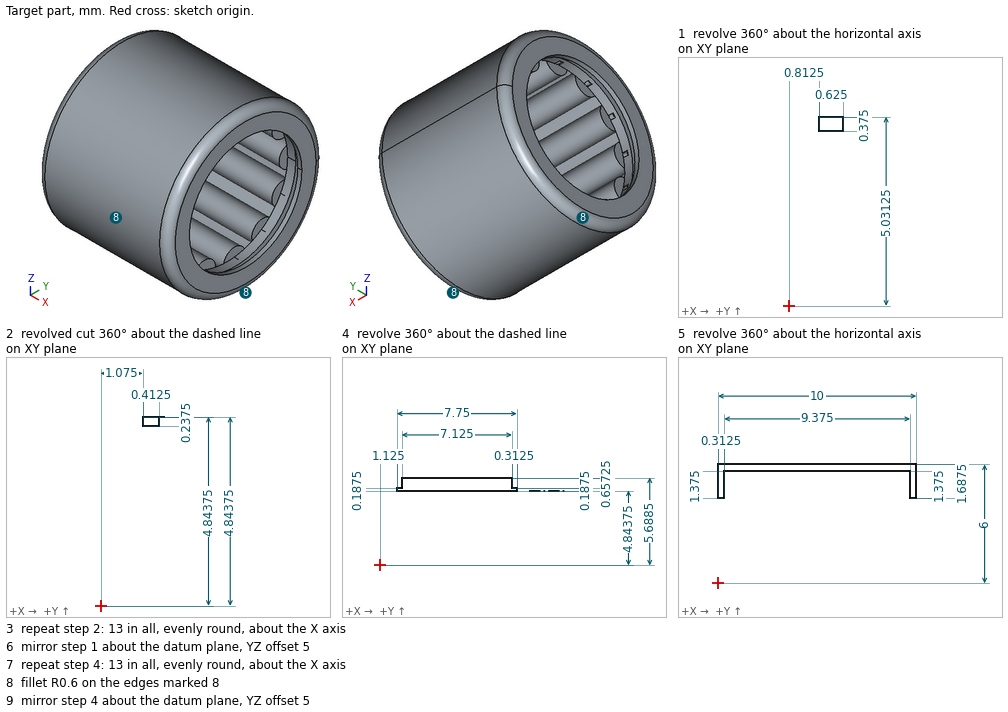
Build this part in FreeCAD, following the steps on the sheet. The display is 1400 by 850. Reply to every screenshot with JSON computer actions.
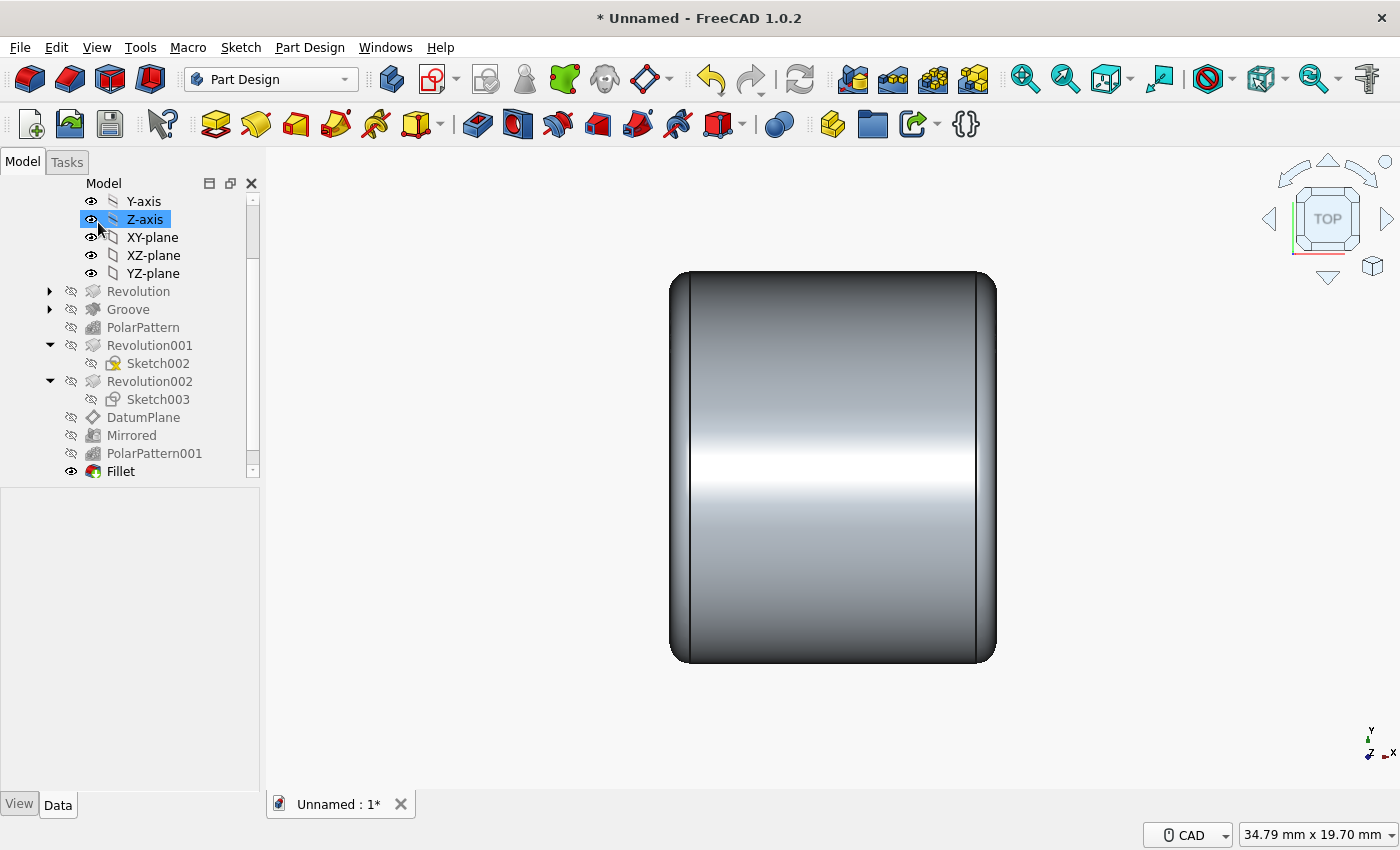
{"action": "scroll", "coordinate": [160, 341], "scroll_direction": "down", "scroll_amount": 3}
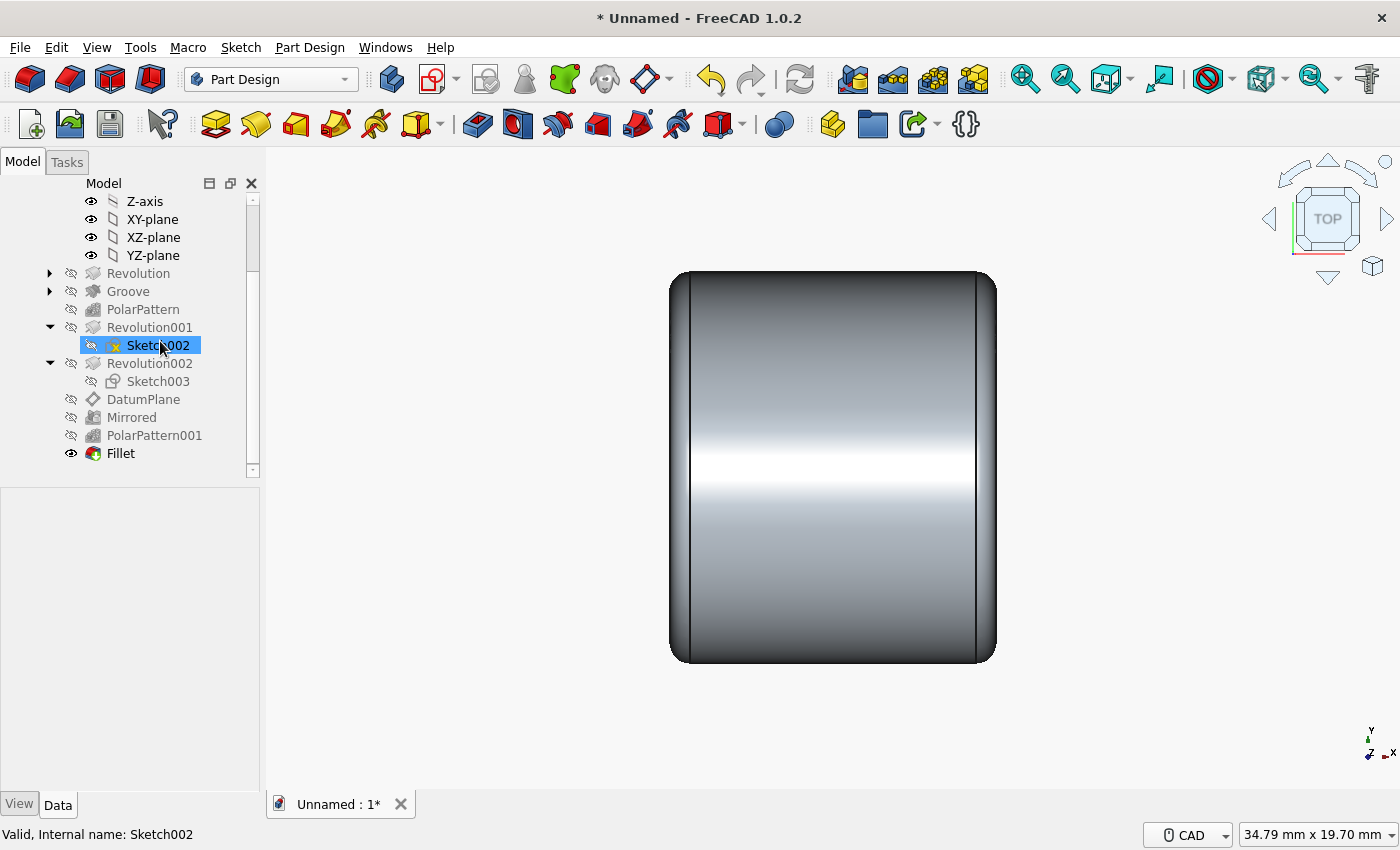
{"action": "scroll", "coordinate": [160, 323], "scroll_direction": "up", "scroll_amount": 15}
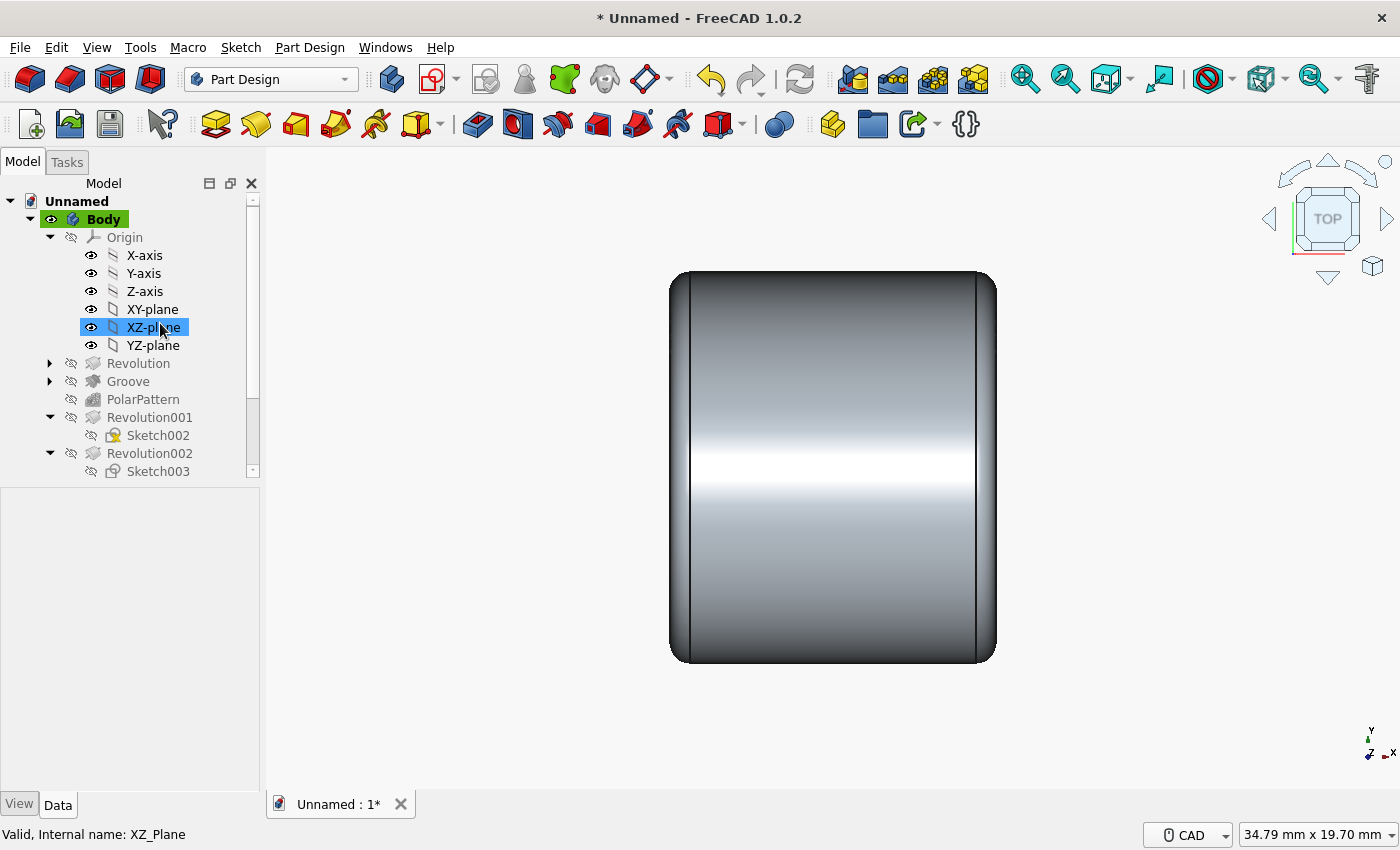
{"action": "left_click", "coordinate": [136, 345]}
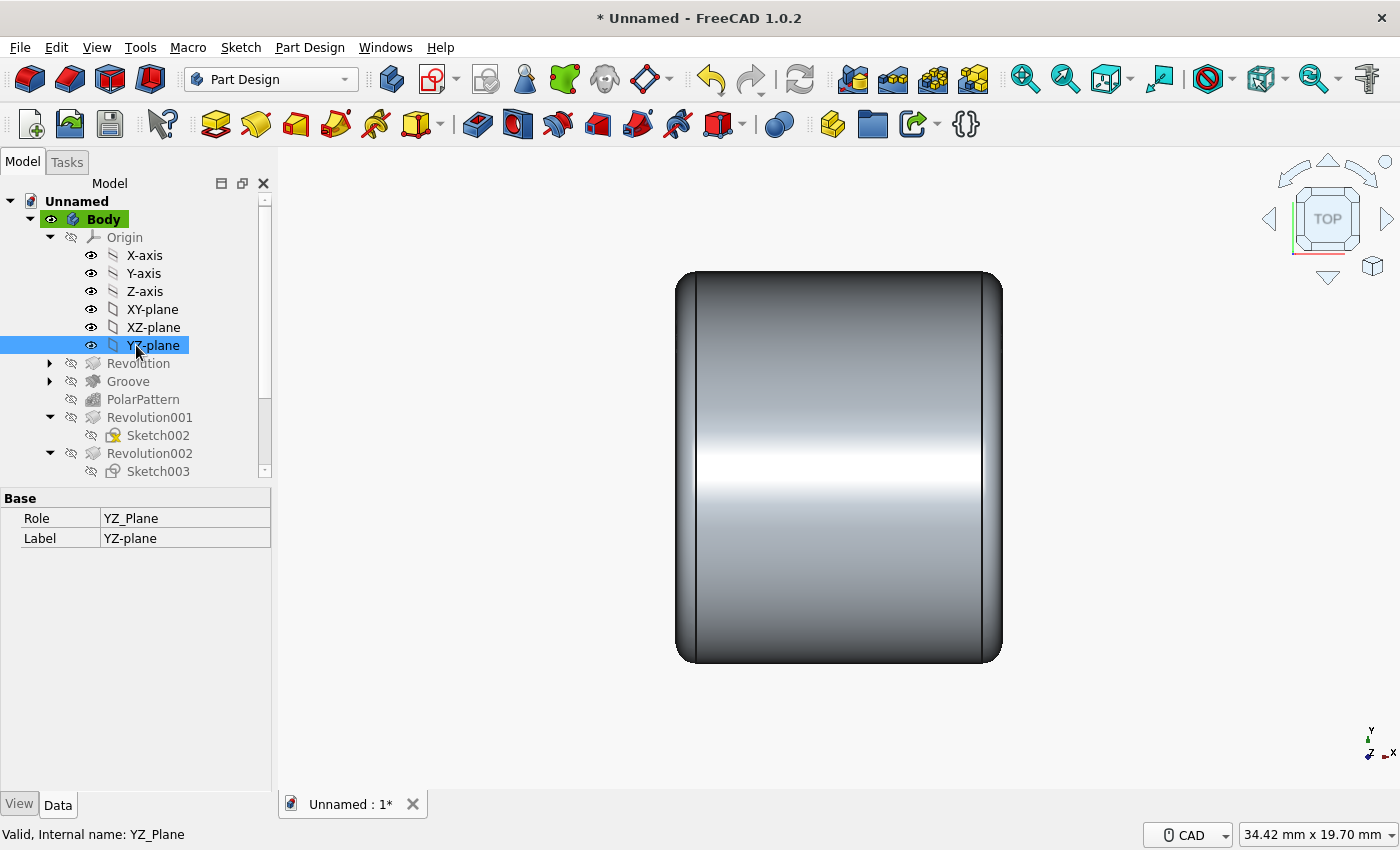
{"action": "left_click", "coordinate": [646, 80]}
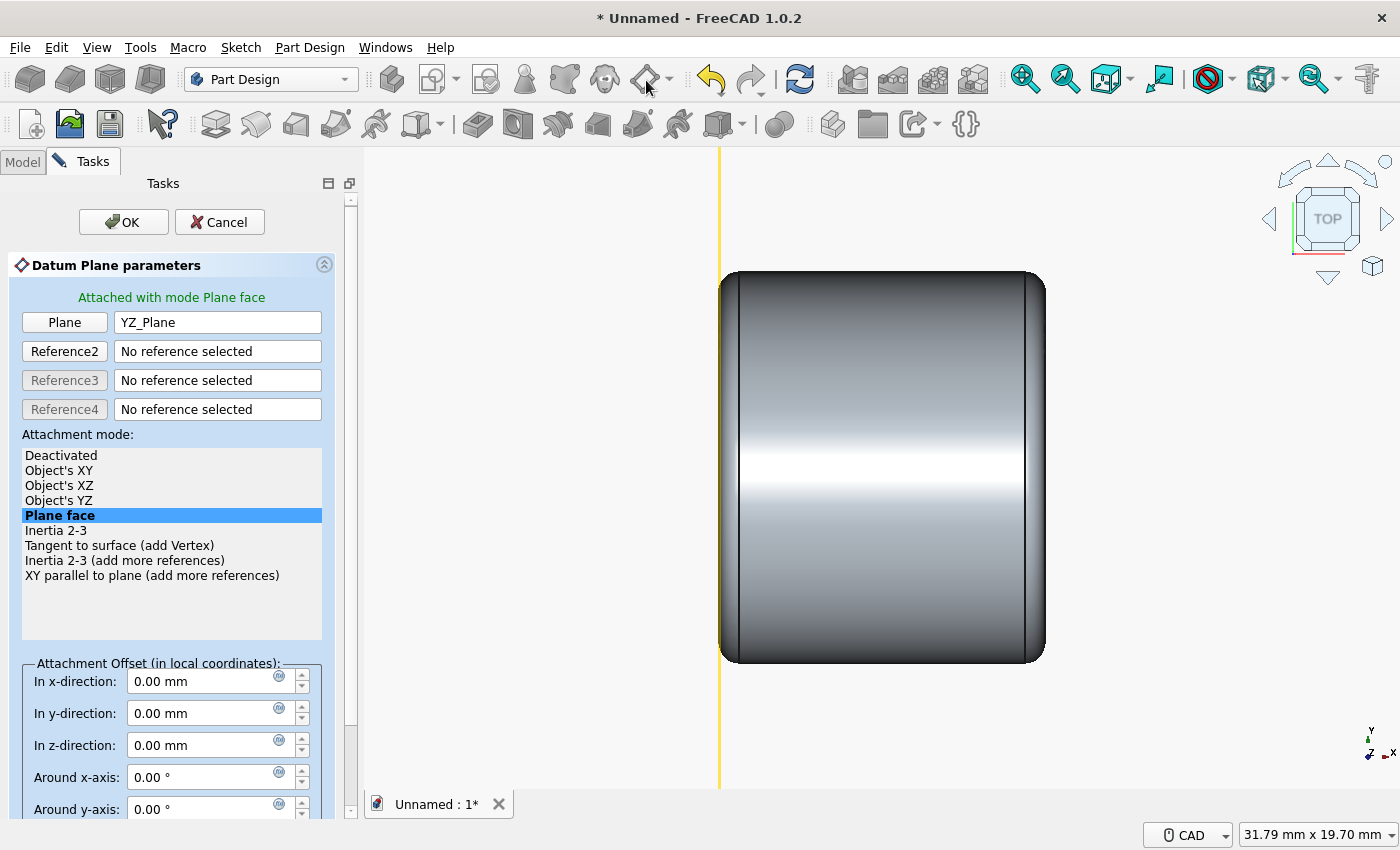
{"action": "triple_click", "coordinate": [210, 745]}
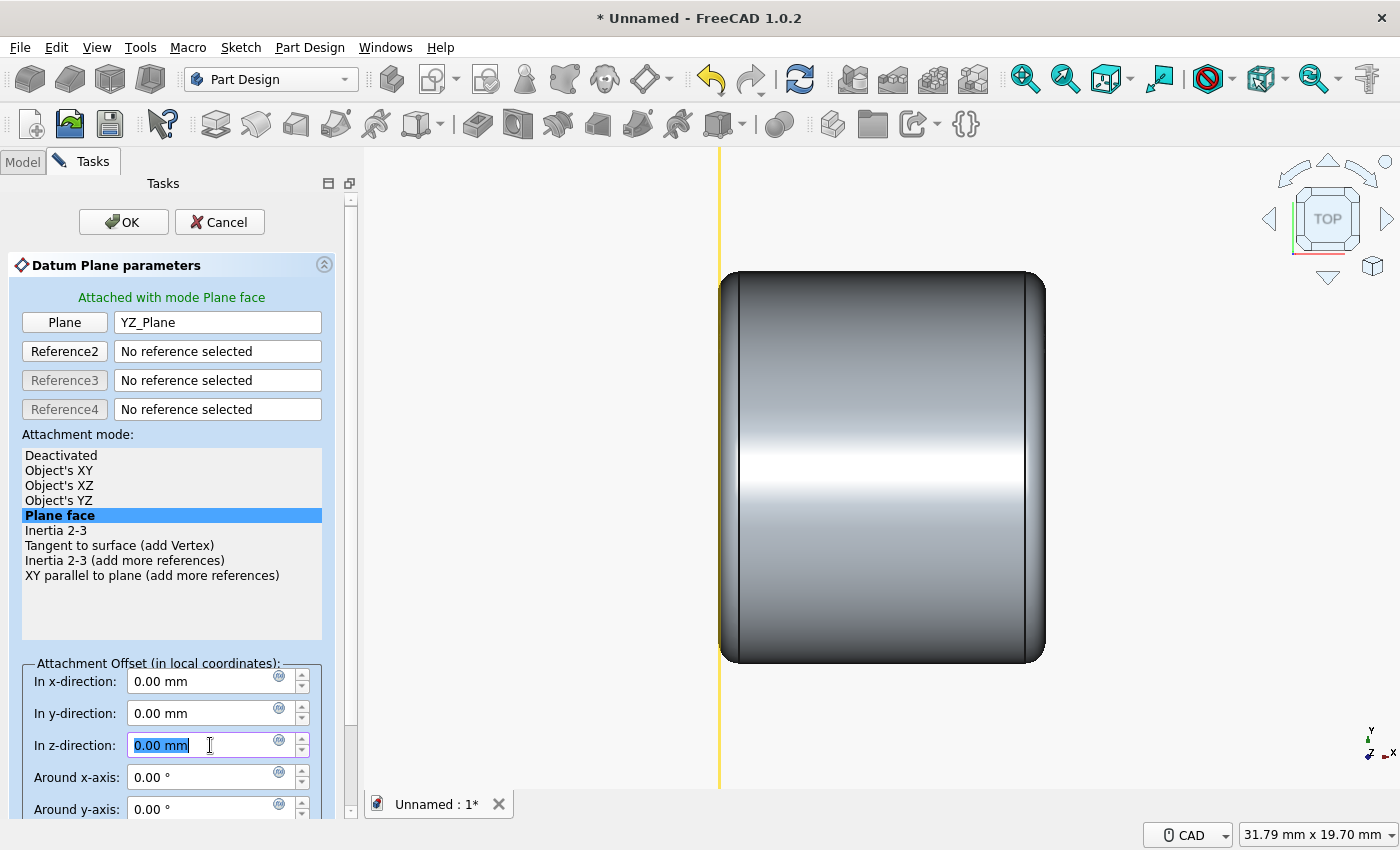
{"action": "type", "text": "5"}
{"action": "key", "text": "Tab"}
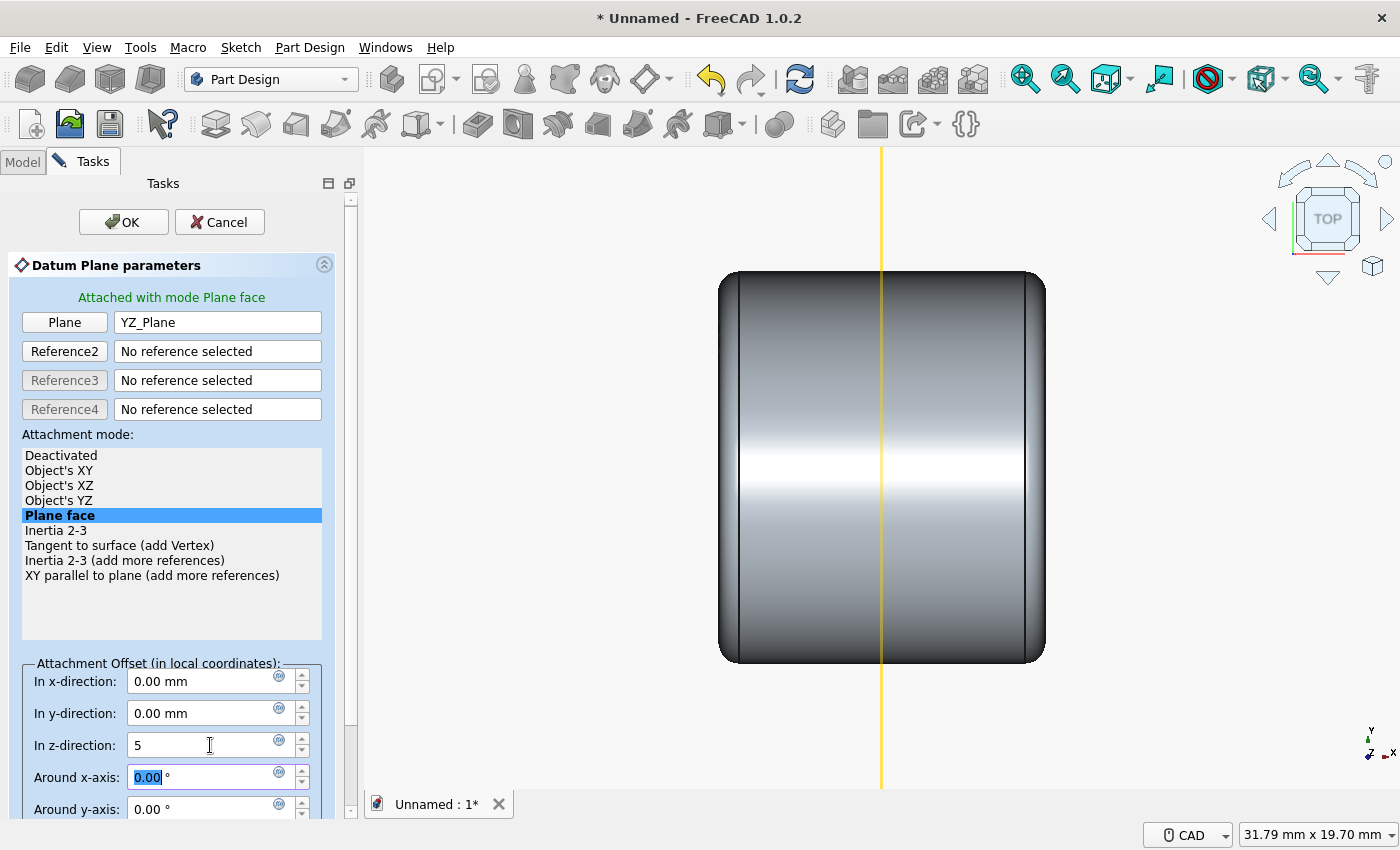
{"action": "left_click", "coordinate": [124, 222]}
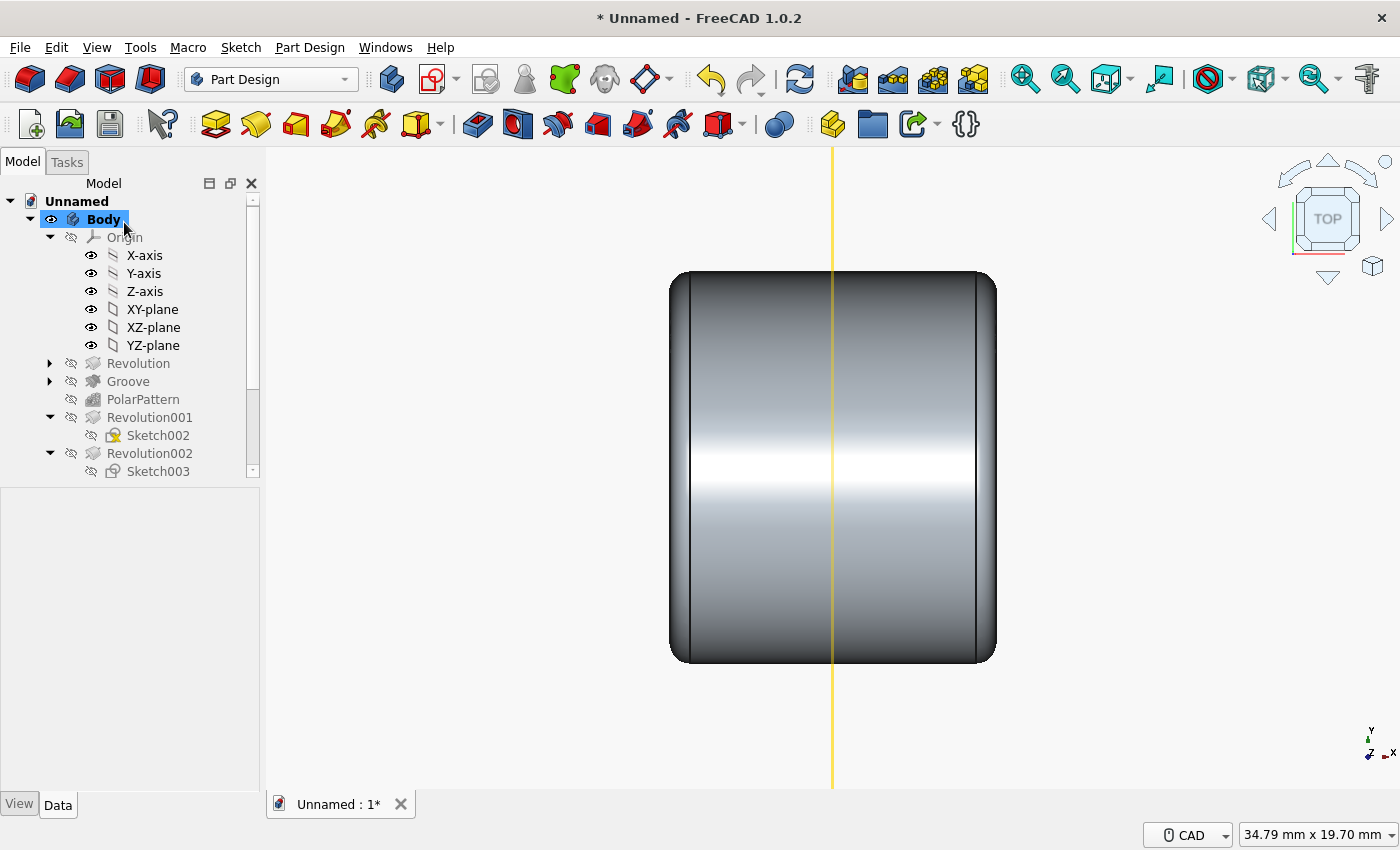
{"action": "left_click", "coordinate": [116, 417]}